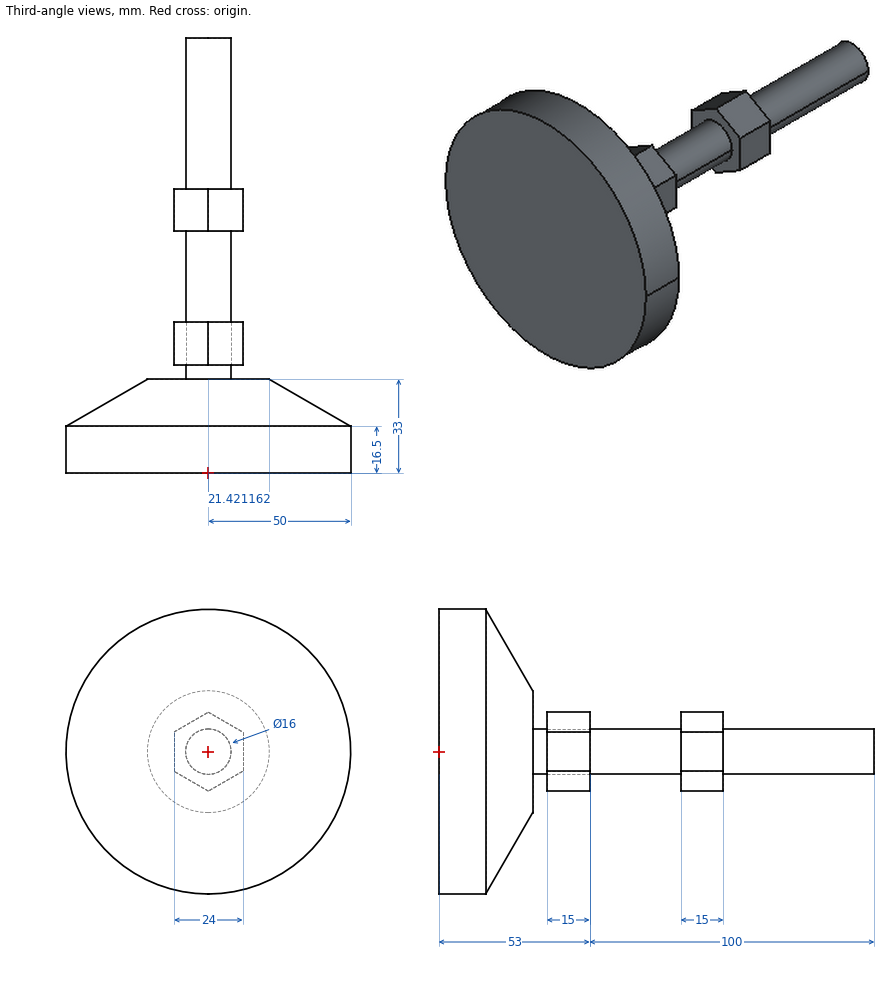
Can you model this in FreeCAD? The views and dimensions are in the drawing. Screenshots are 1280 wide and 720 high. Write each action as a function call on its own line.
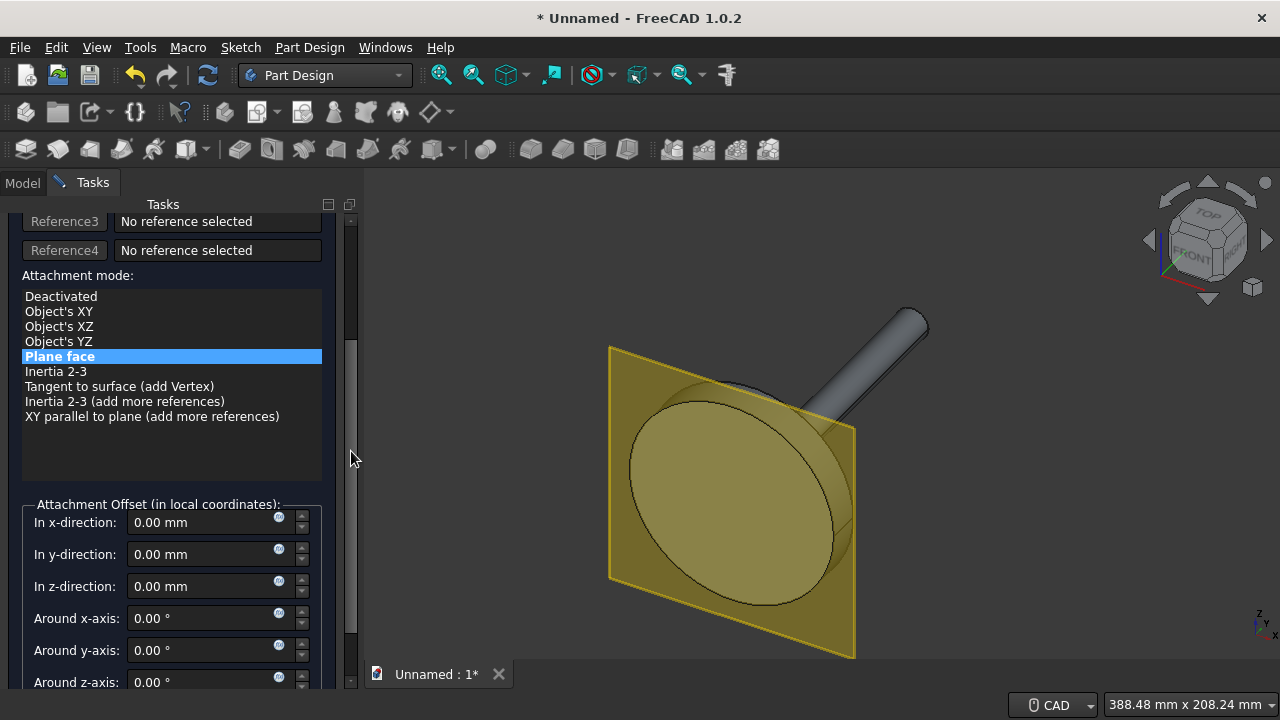
triple_click(210, 586)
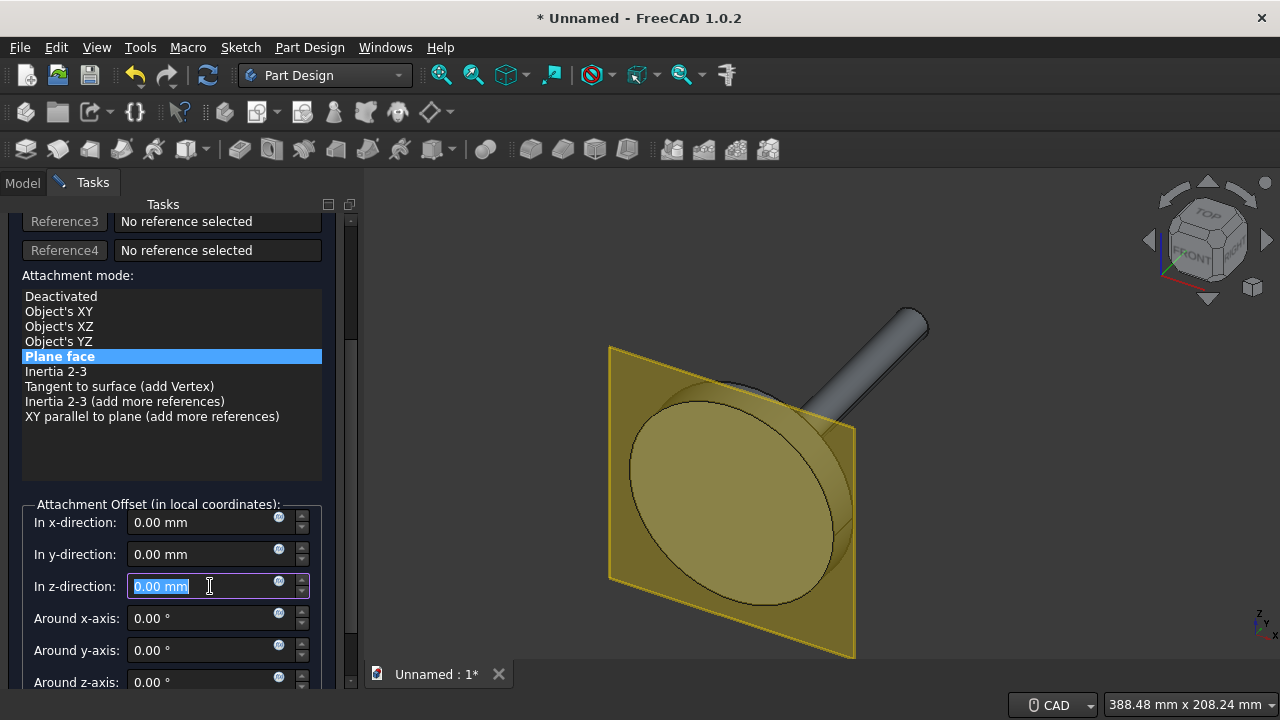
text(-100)
key(Tab)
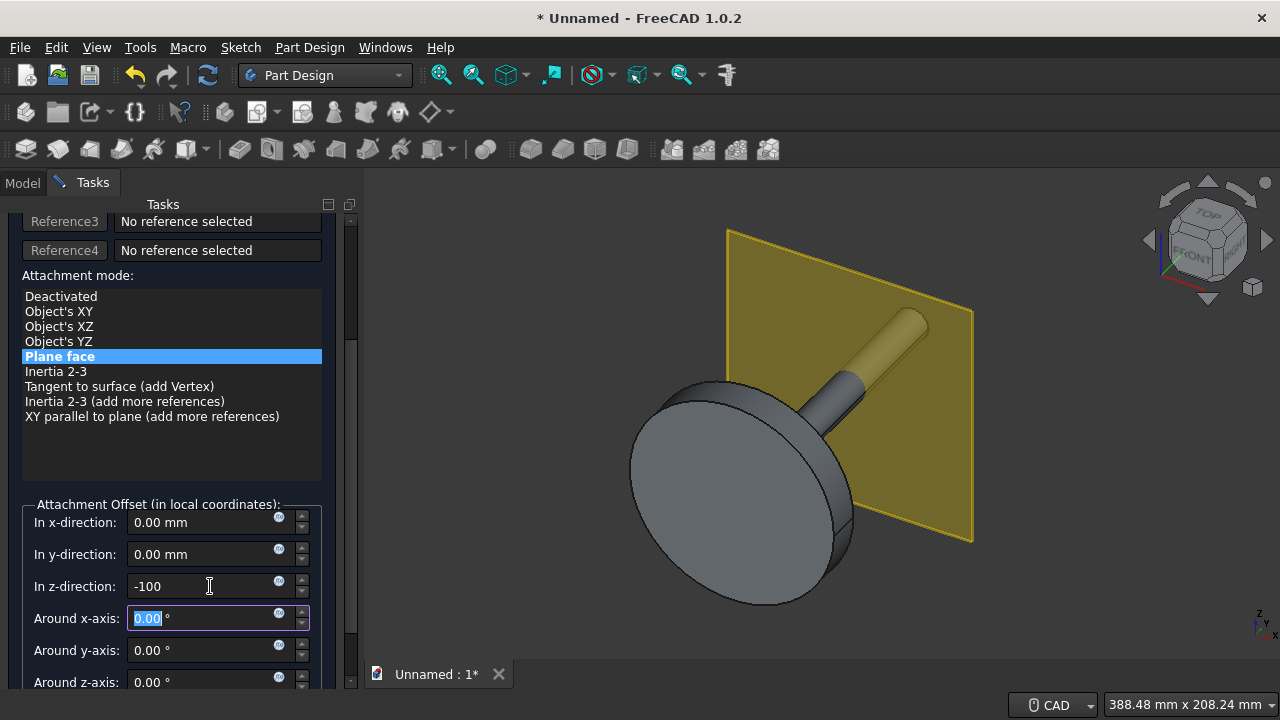
scroll(351, 451, up, 4)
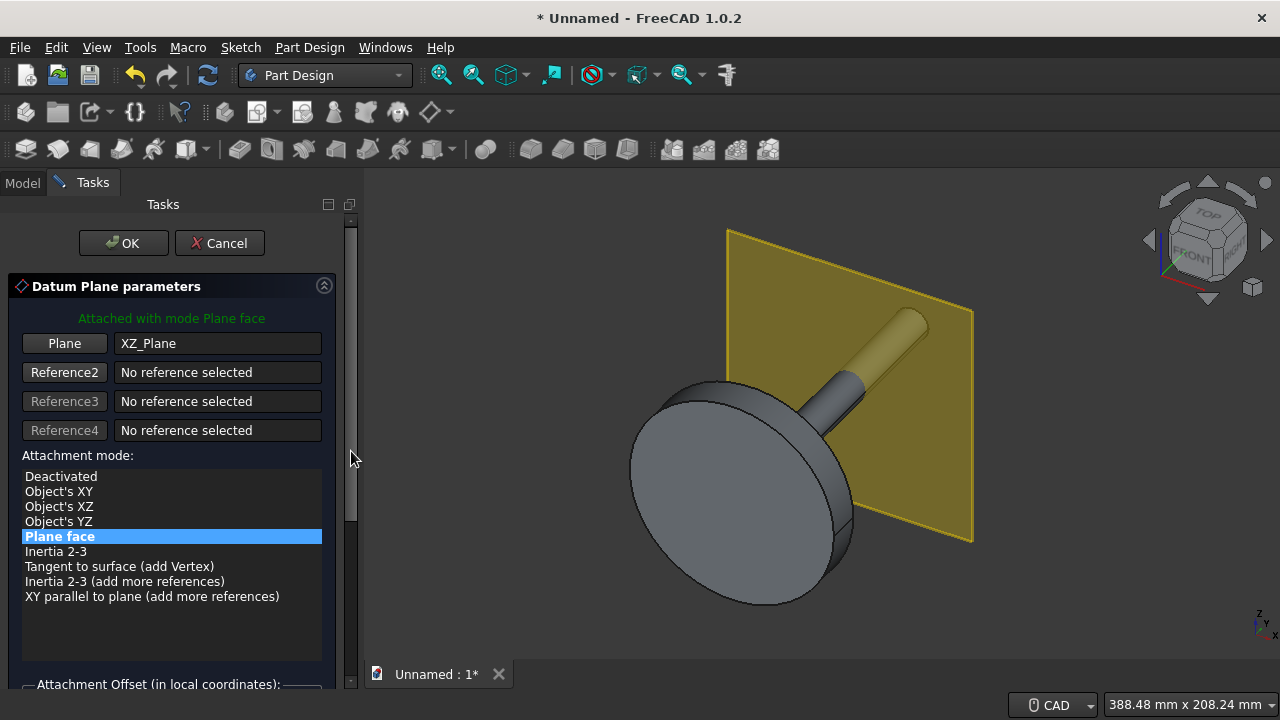
click(124, 243)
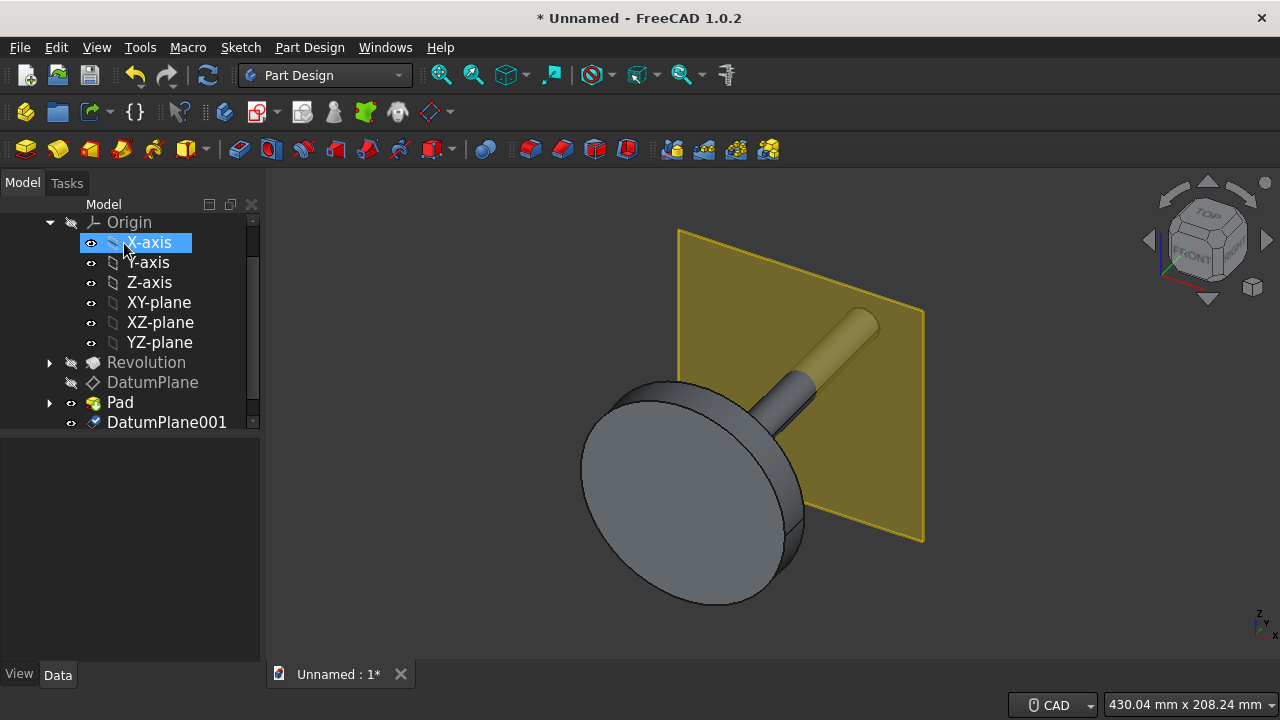
click(116, 423)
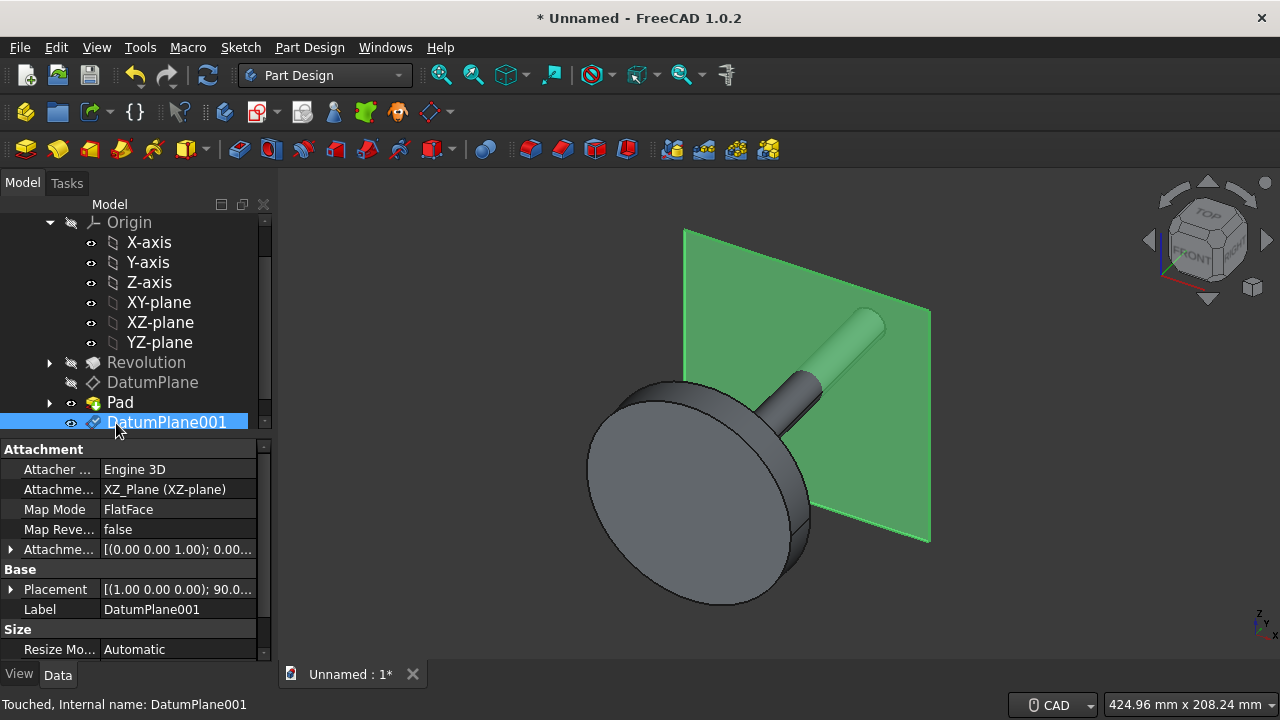
click(258, 112)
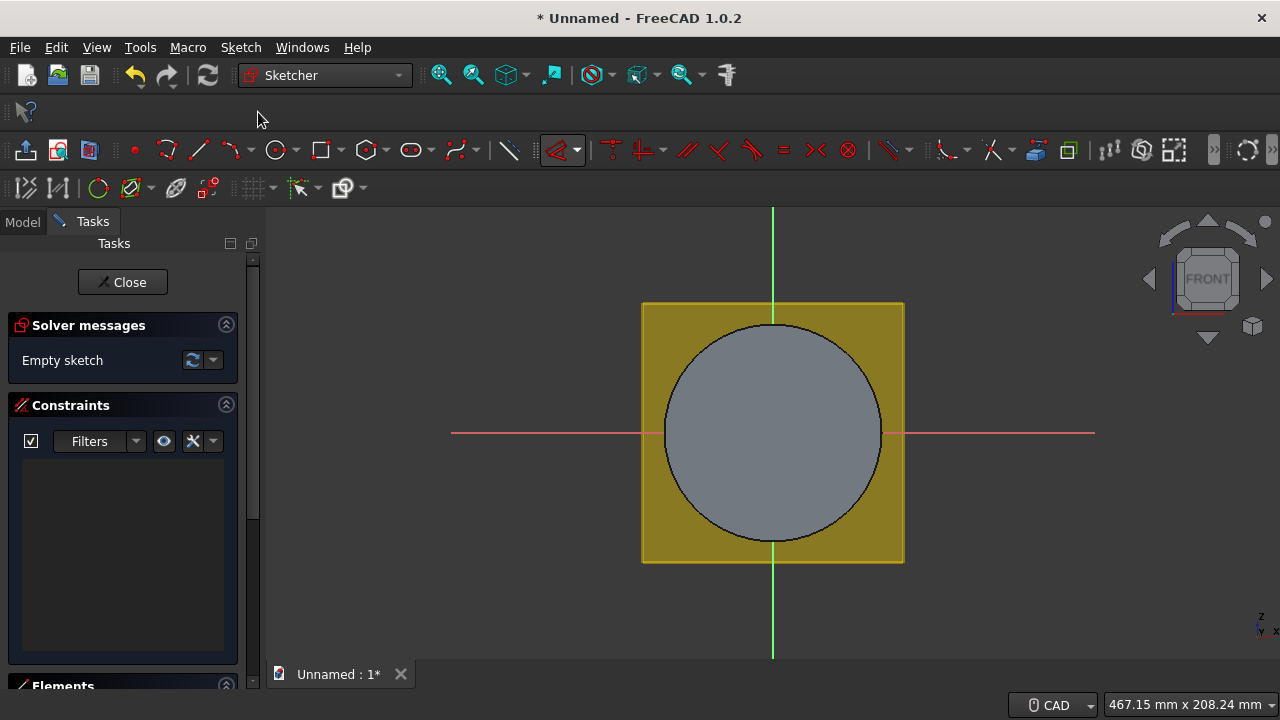
click(90, 150)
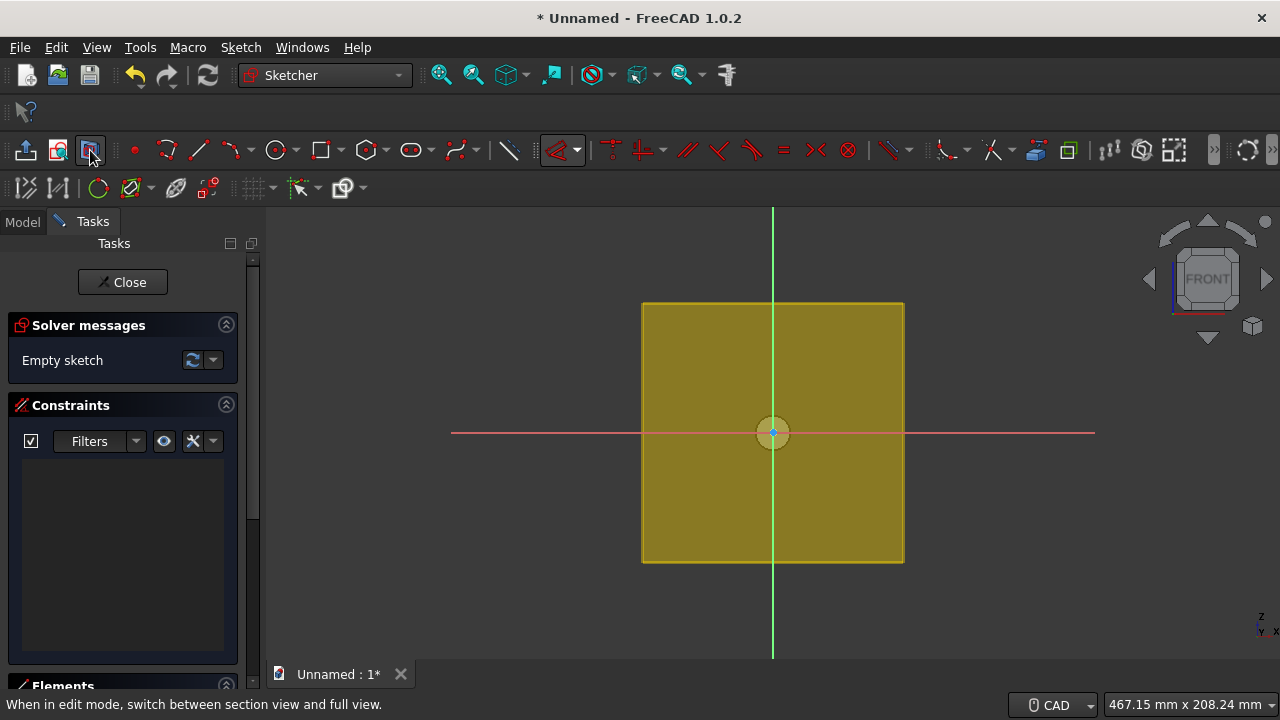
scroll(790, 433, up, 8)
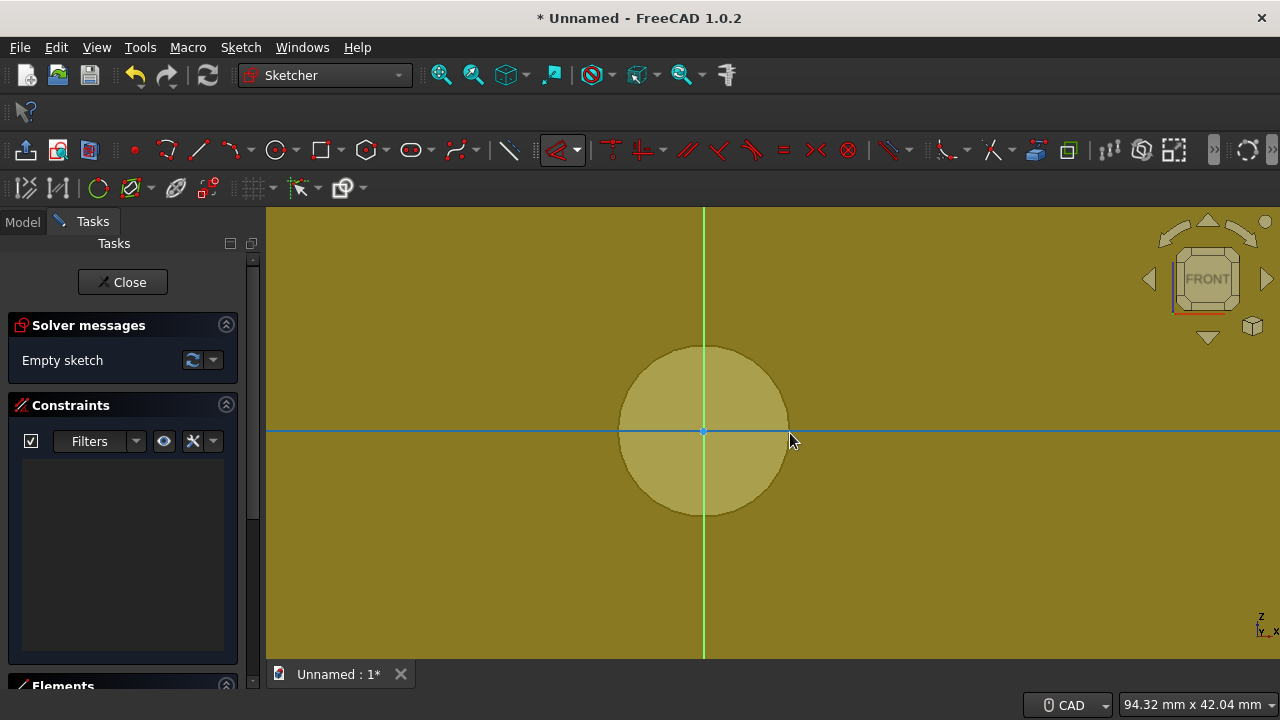
click(366, 150)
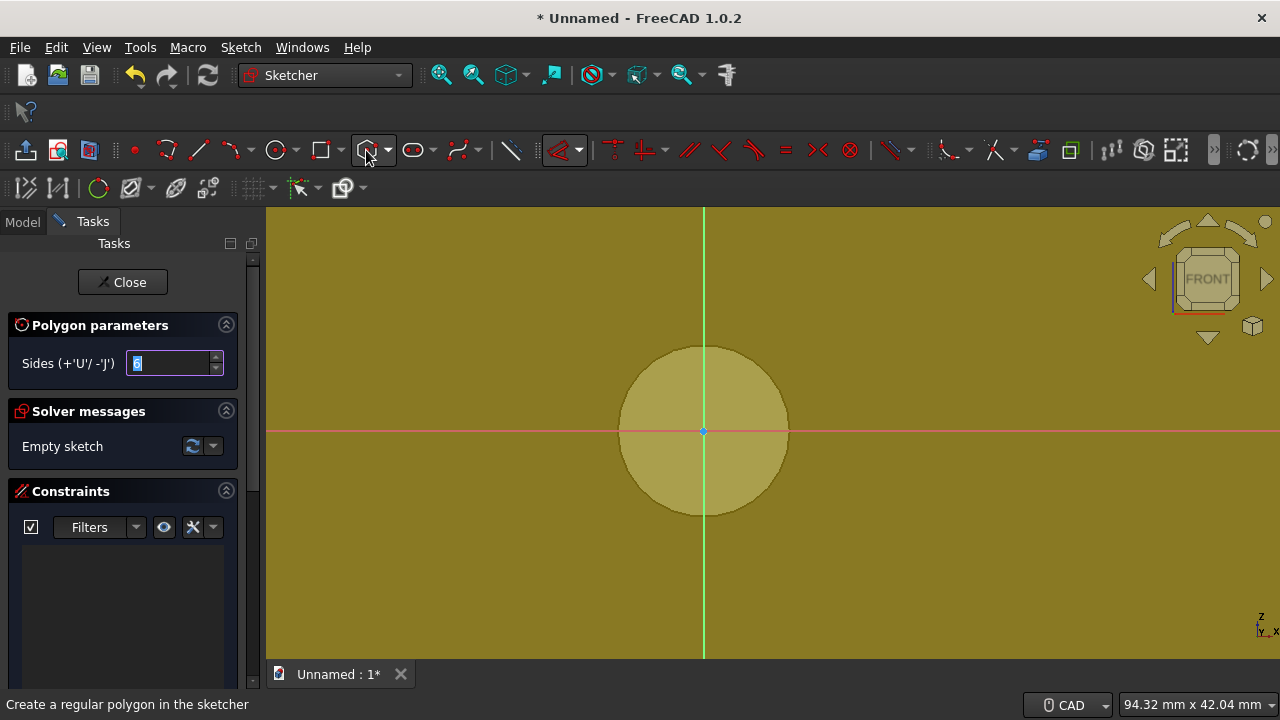
click(704, 431)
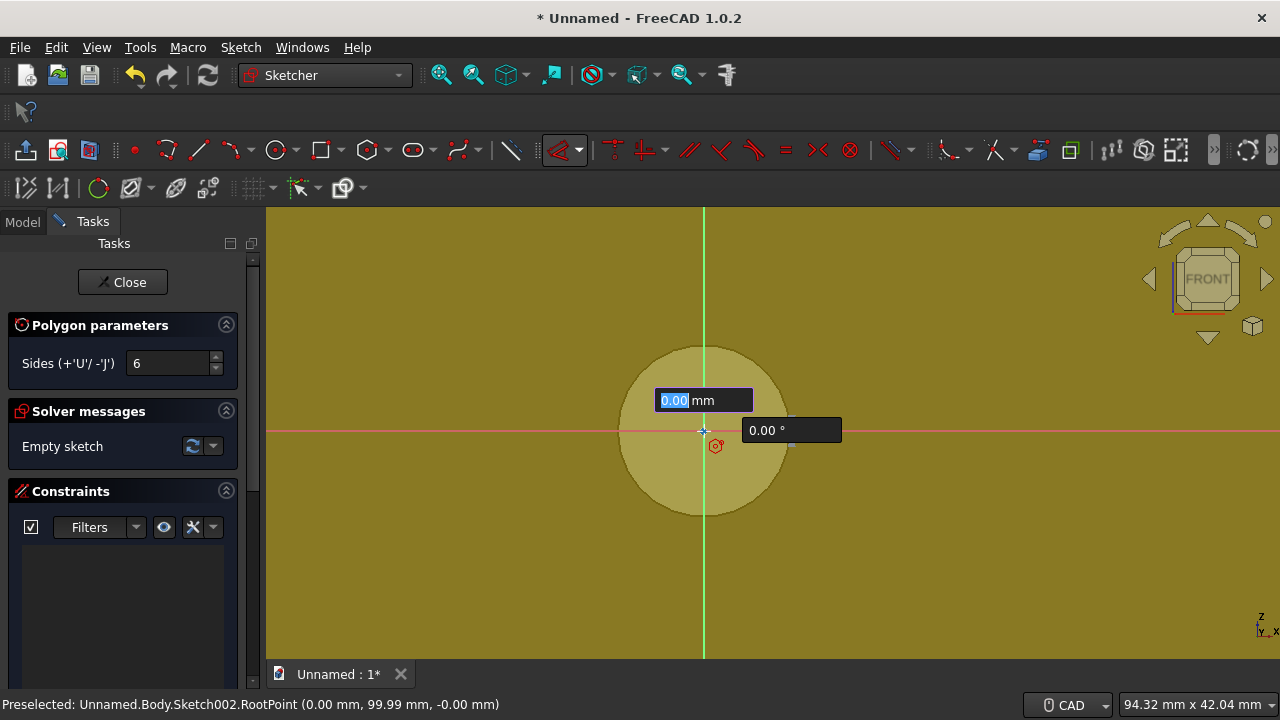
click(704, 282)
key(Escape)